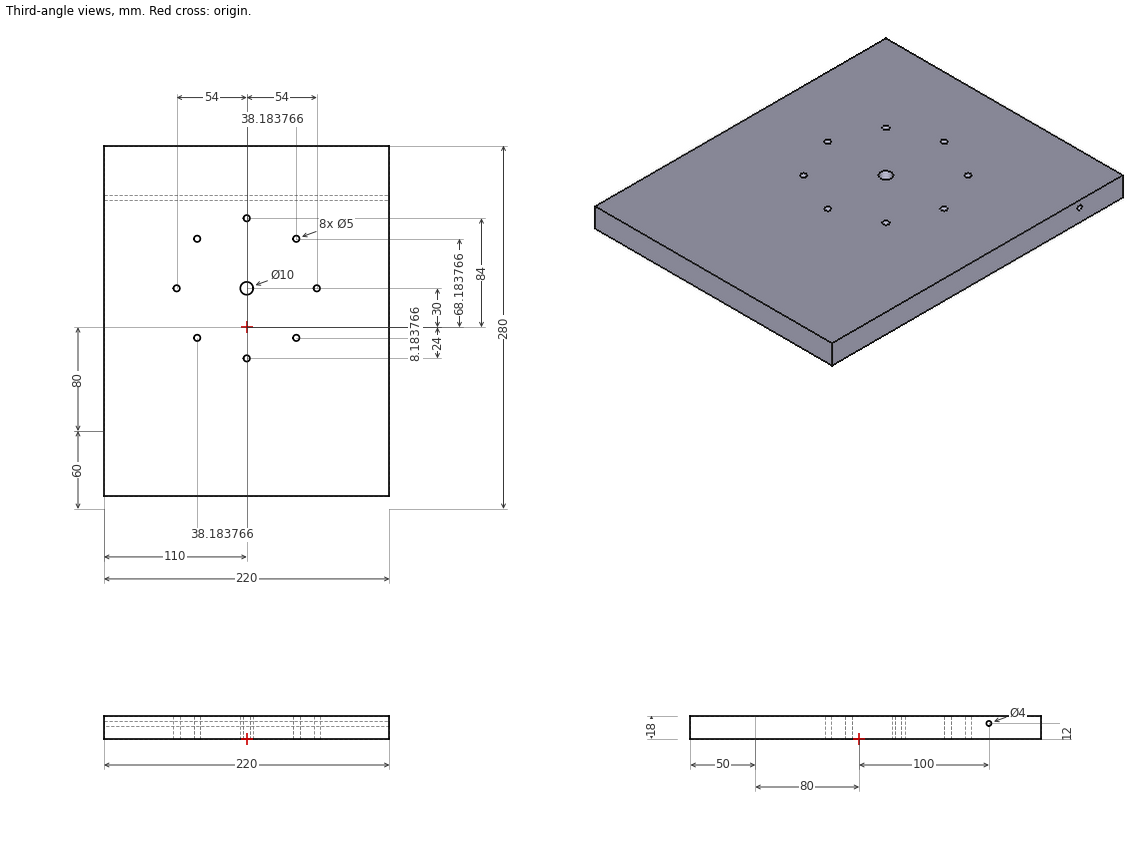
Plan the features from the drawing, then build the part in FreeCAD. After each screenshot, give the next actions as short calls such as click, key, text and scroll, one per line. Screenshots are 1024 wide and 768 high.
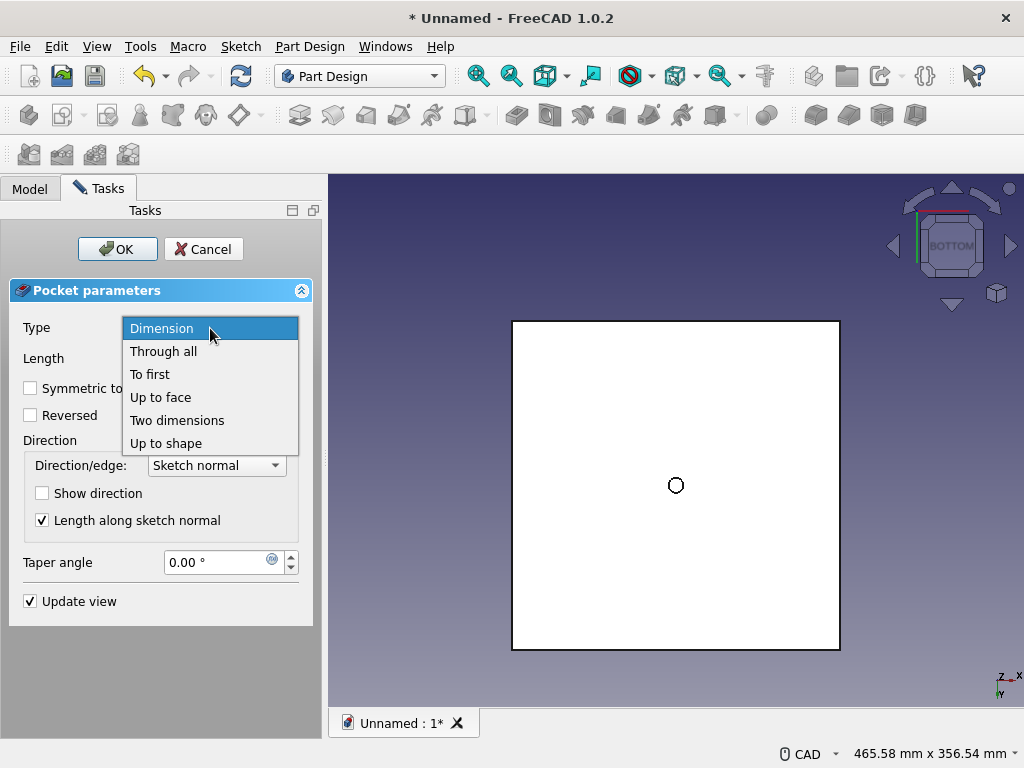
click(208, 352)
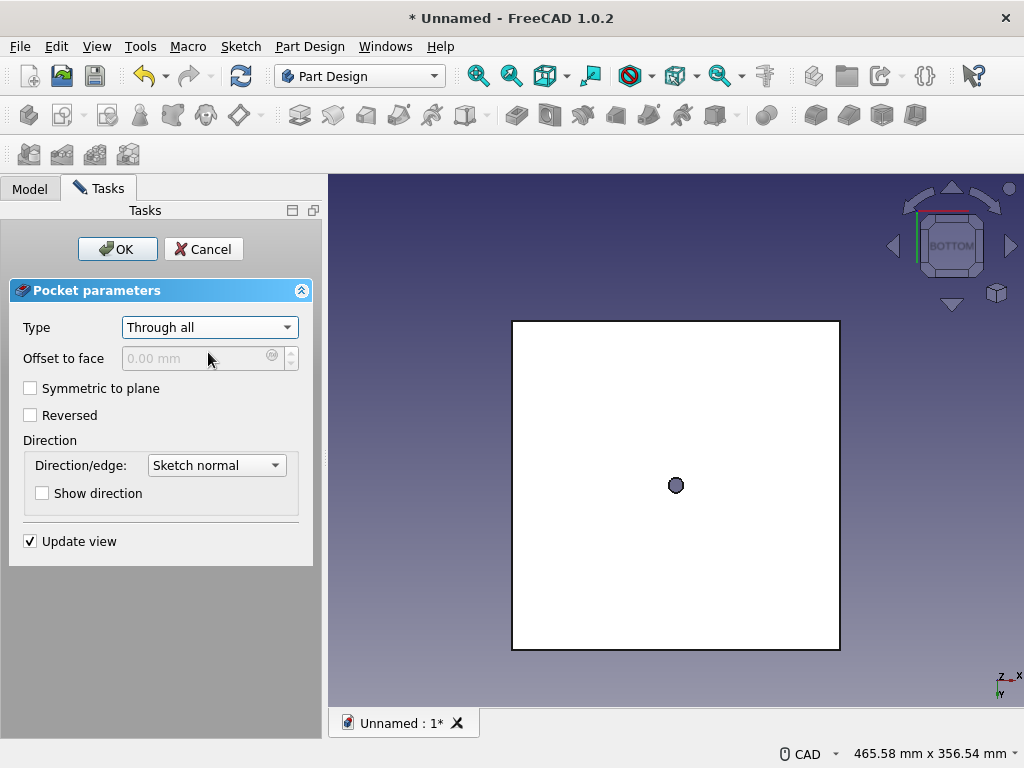
click(118, 249)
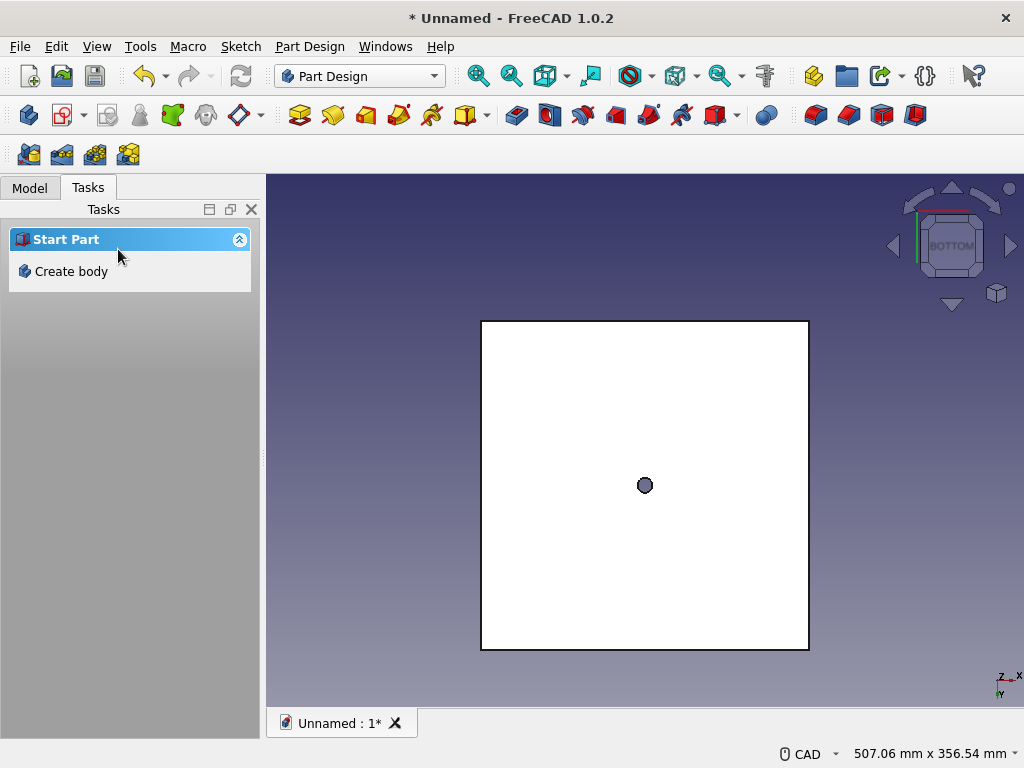
click(692, 390)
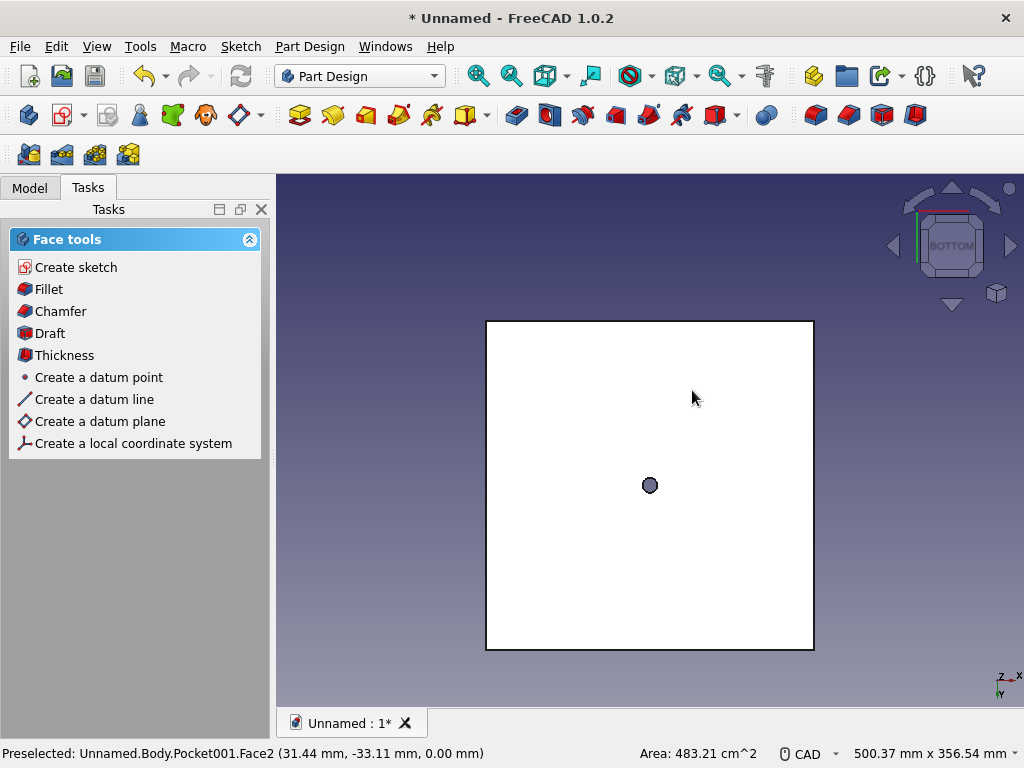
click(62, 116)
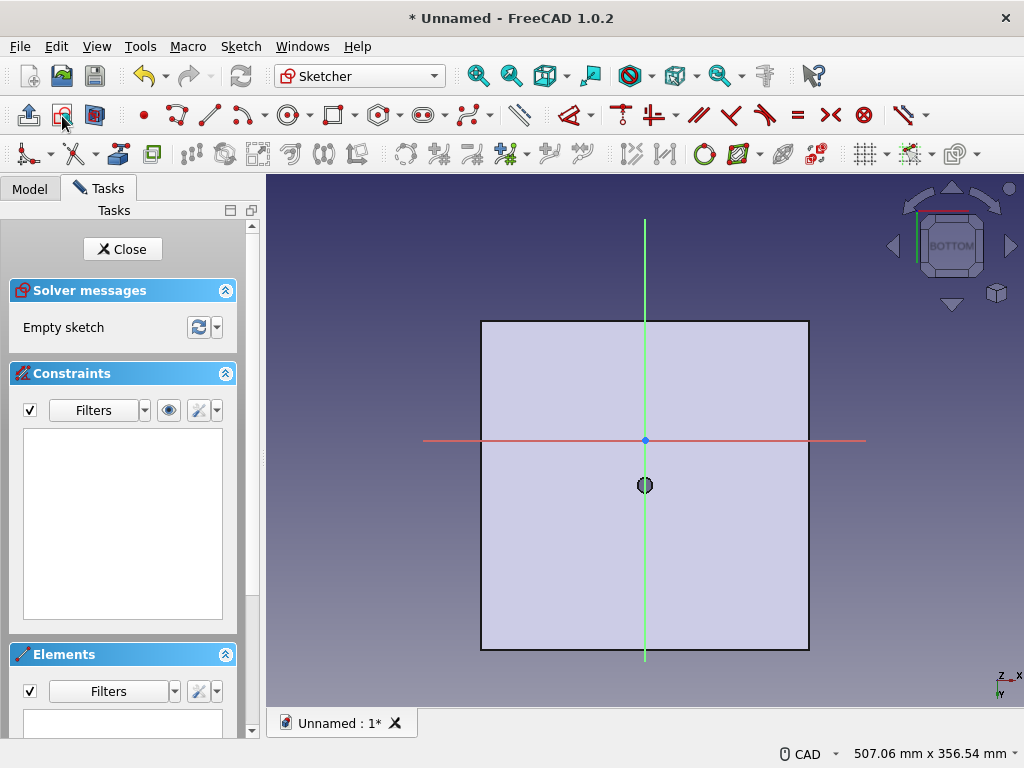
scroll(728, 540, up, 3)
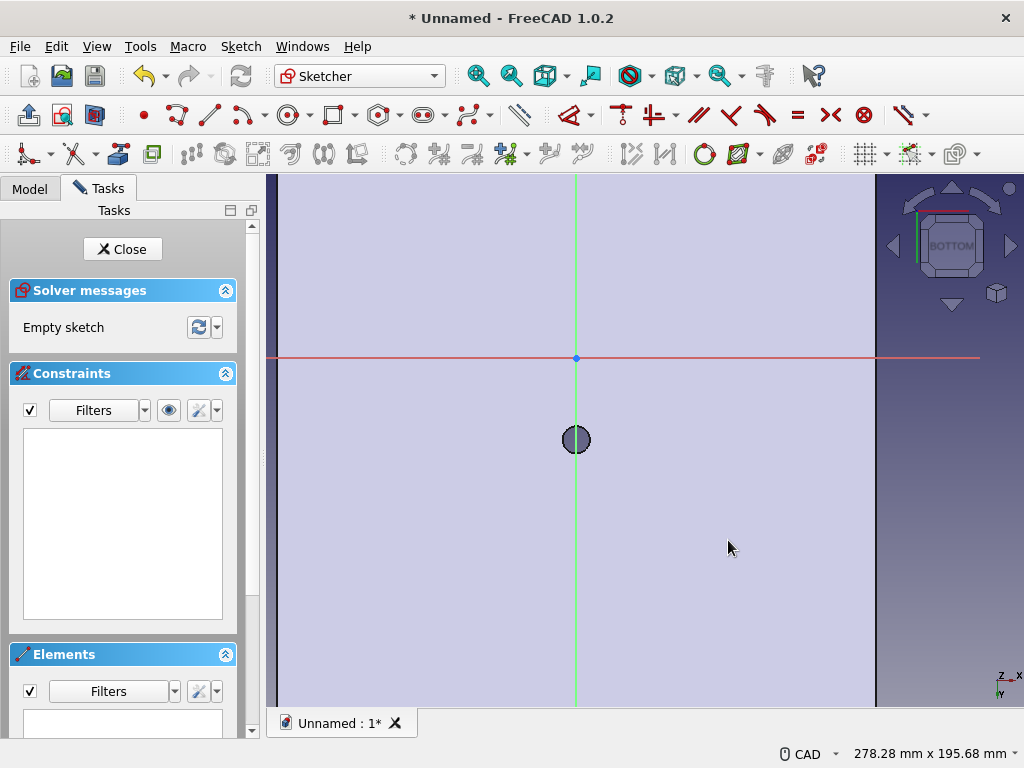
click(288, 116)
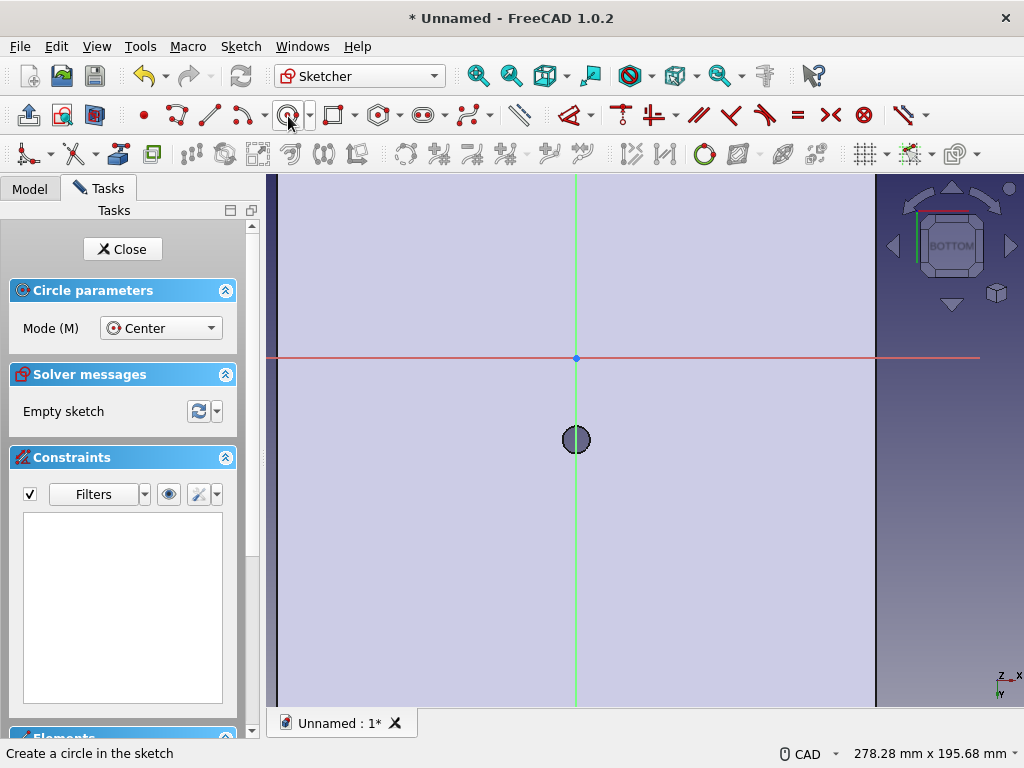
scroll(680, 544, up, 7)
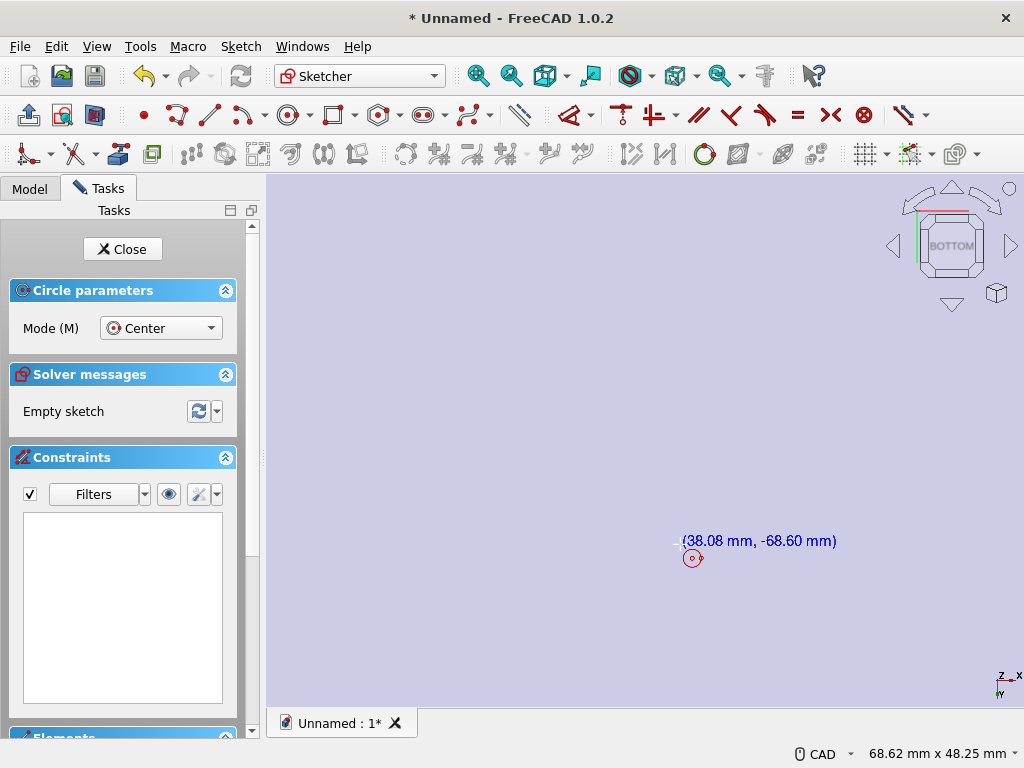
scroll(681, 546, down, 7)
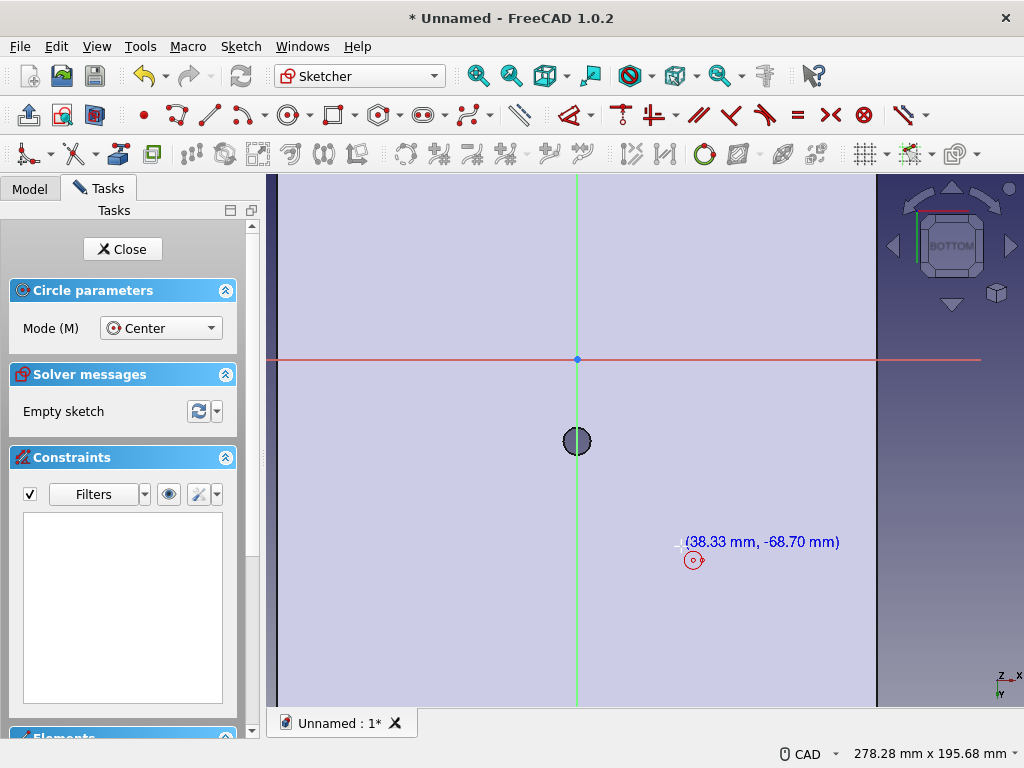
click(681, 545)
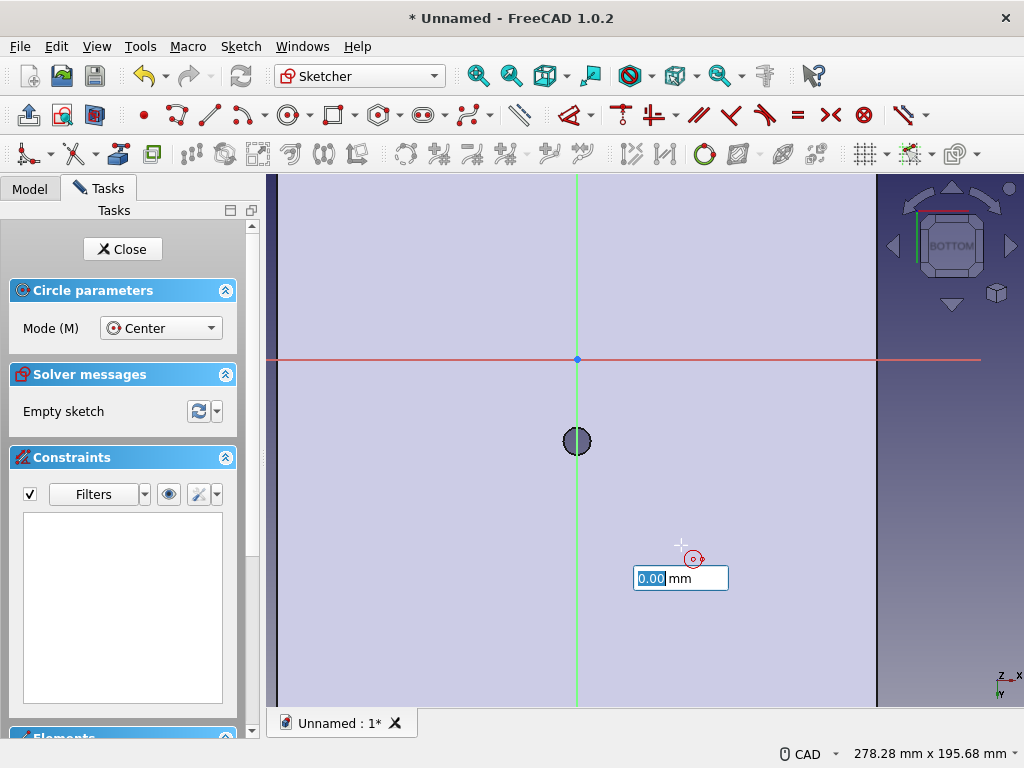
scroll(686, 541, up, 5)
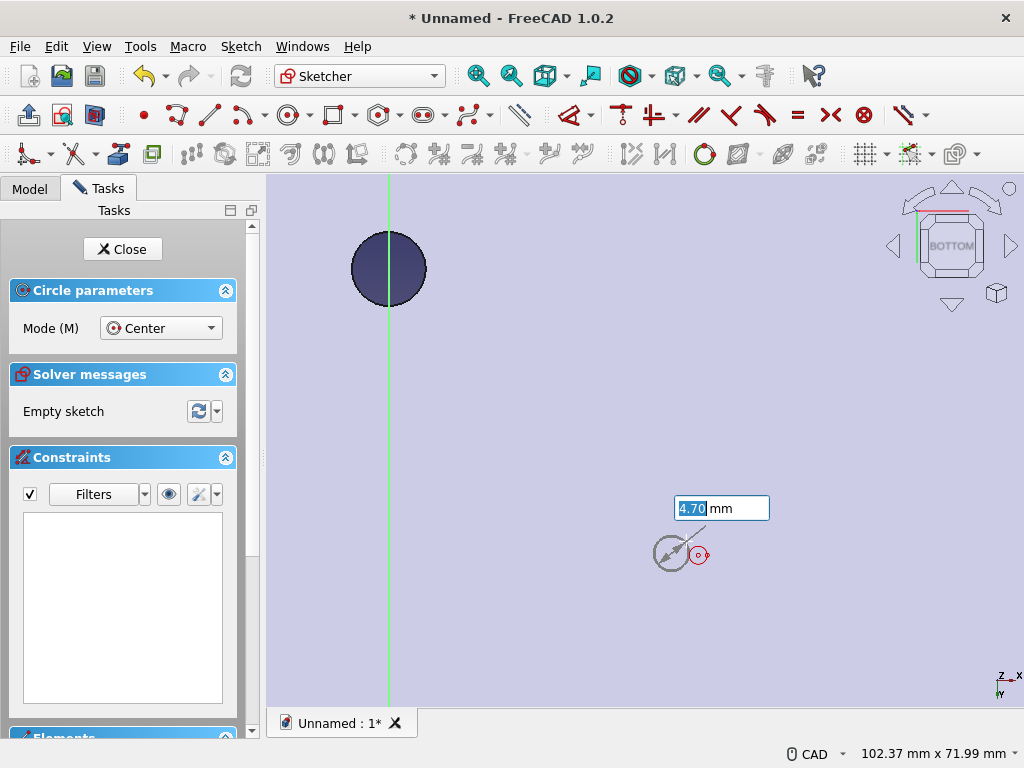
click(685, 539)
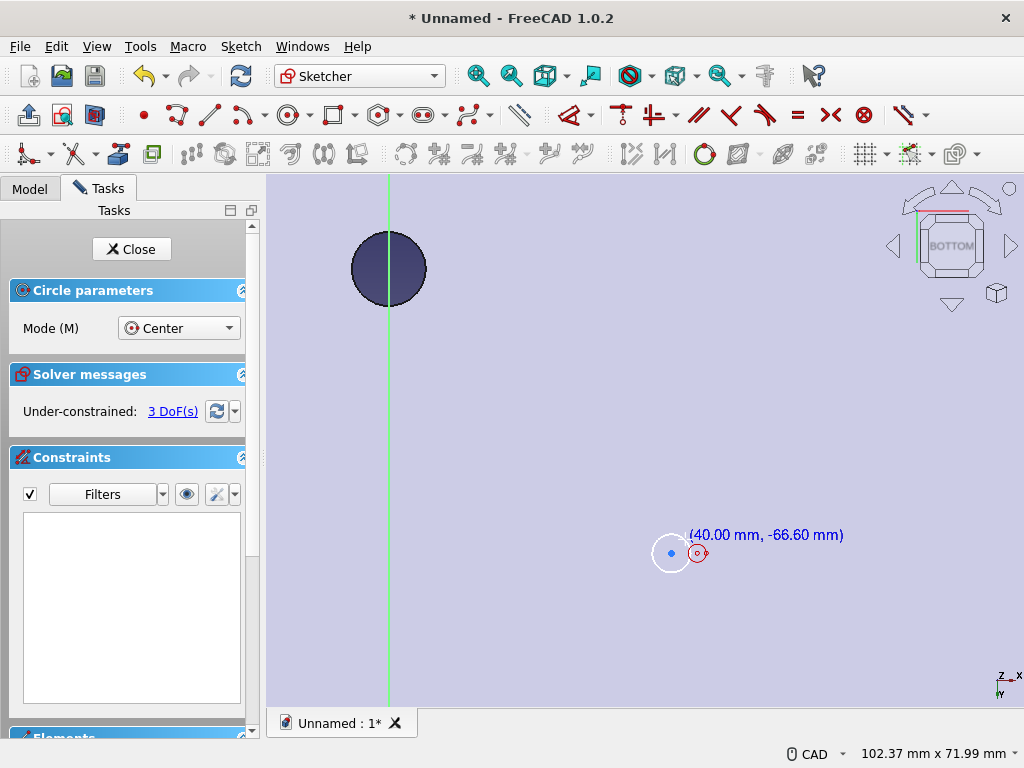
scroll(389, 669, up, 2)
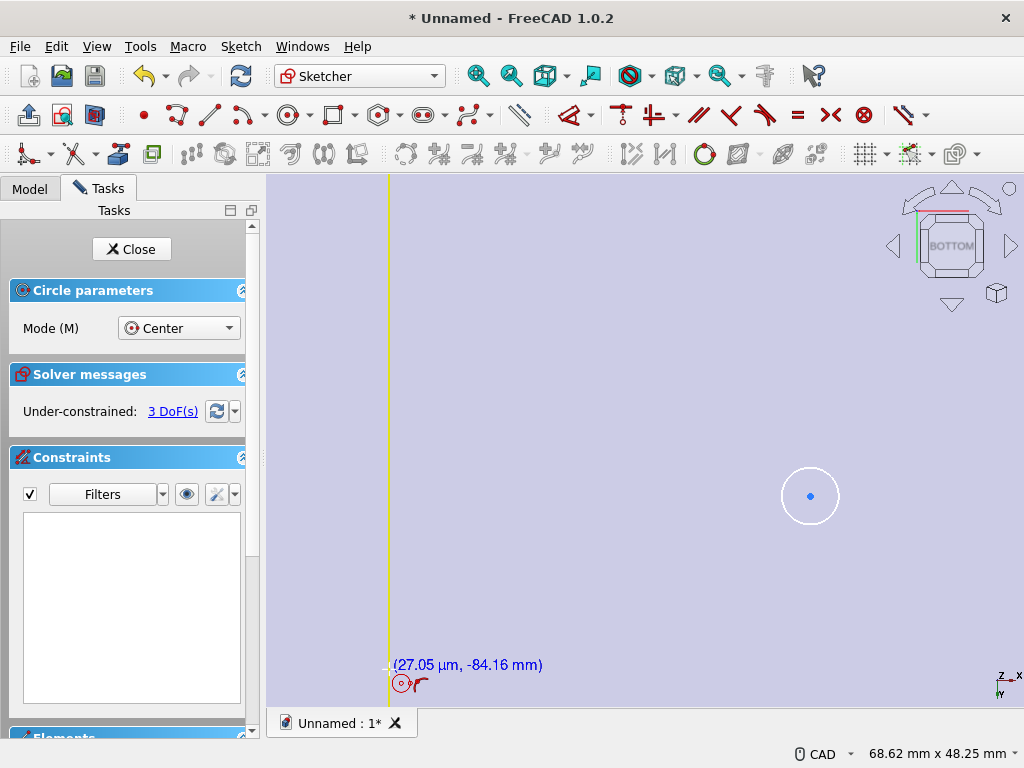
scroll(638, 561, down, 7)